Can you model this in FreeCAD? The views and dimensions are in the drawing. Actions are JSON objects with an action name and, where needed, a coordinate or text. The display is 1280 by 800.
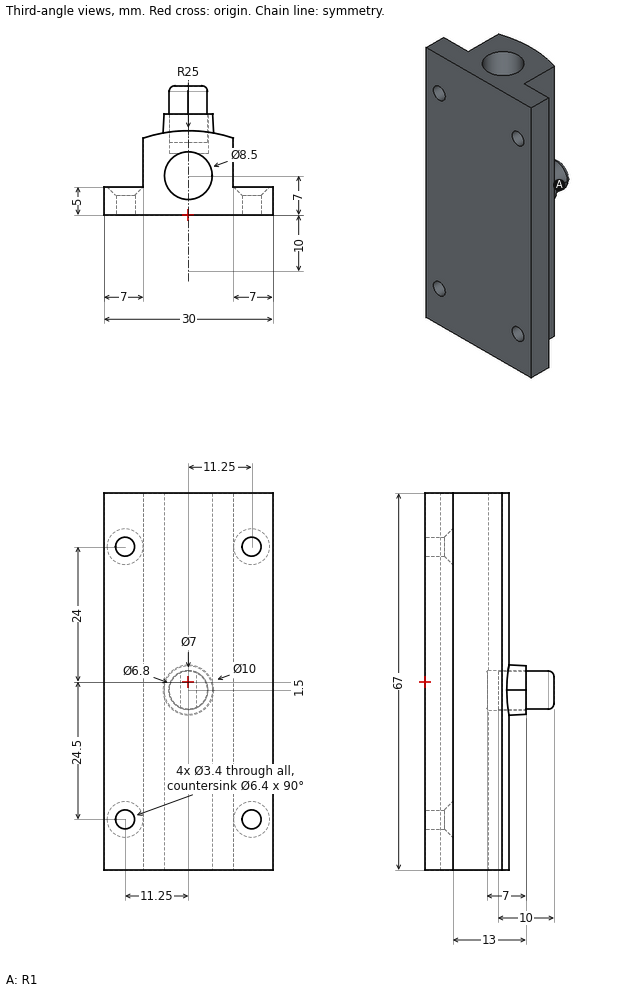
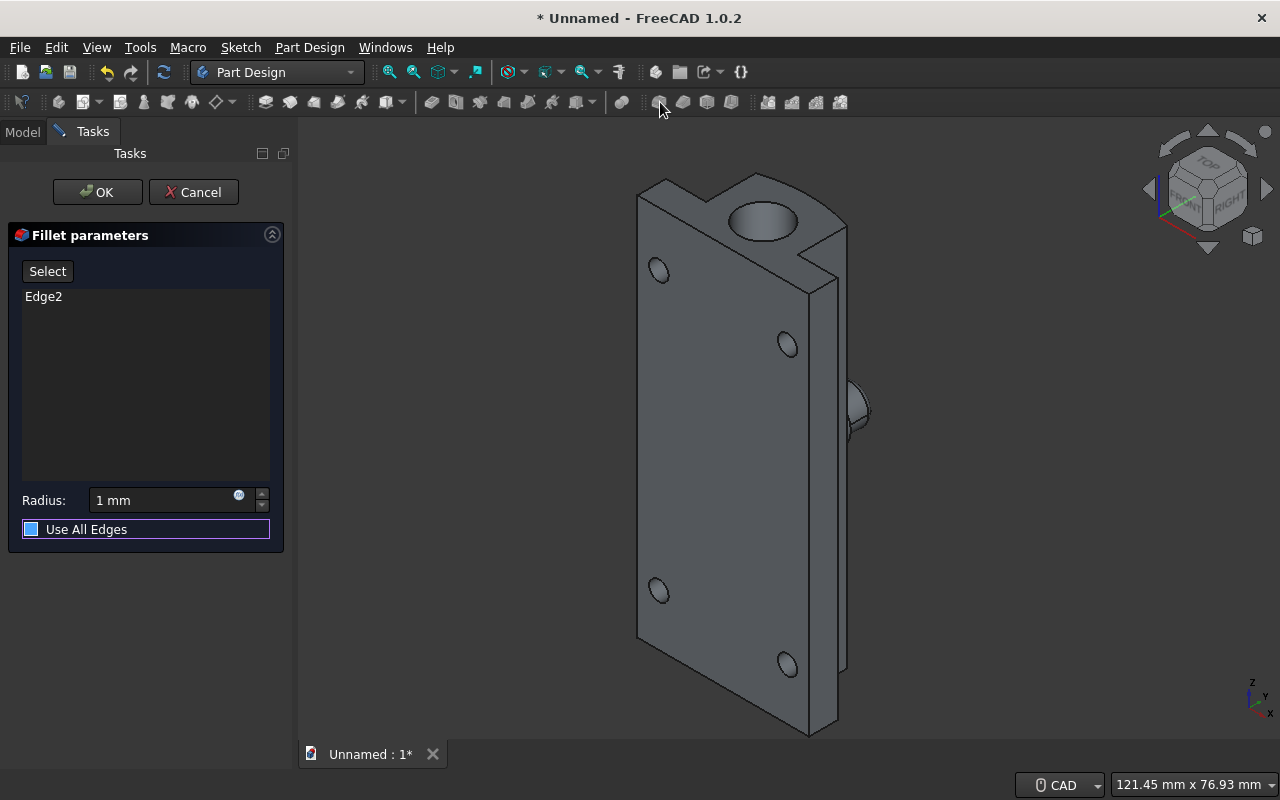
{"action": "left_click", "coordinate": [98, 192]}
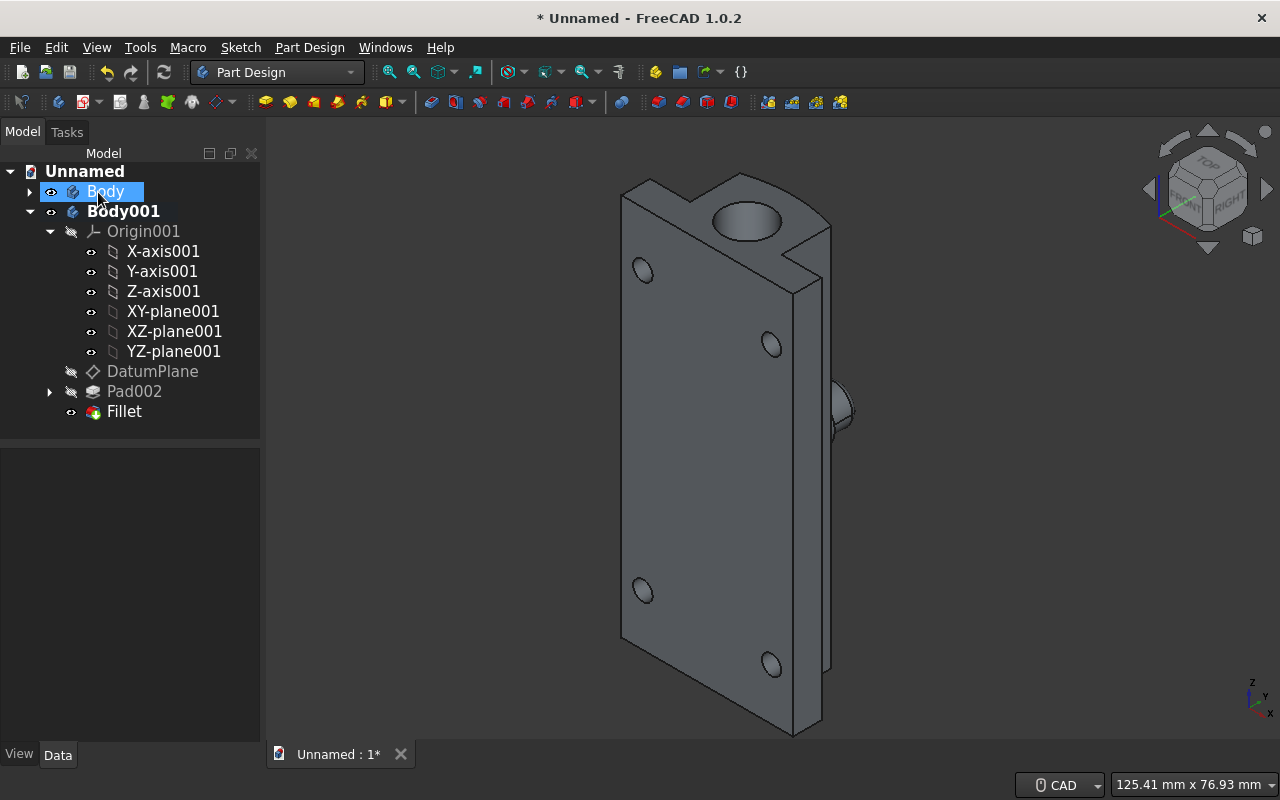
{"action": "left_click", "coordinate": [390, 72]}